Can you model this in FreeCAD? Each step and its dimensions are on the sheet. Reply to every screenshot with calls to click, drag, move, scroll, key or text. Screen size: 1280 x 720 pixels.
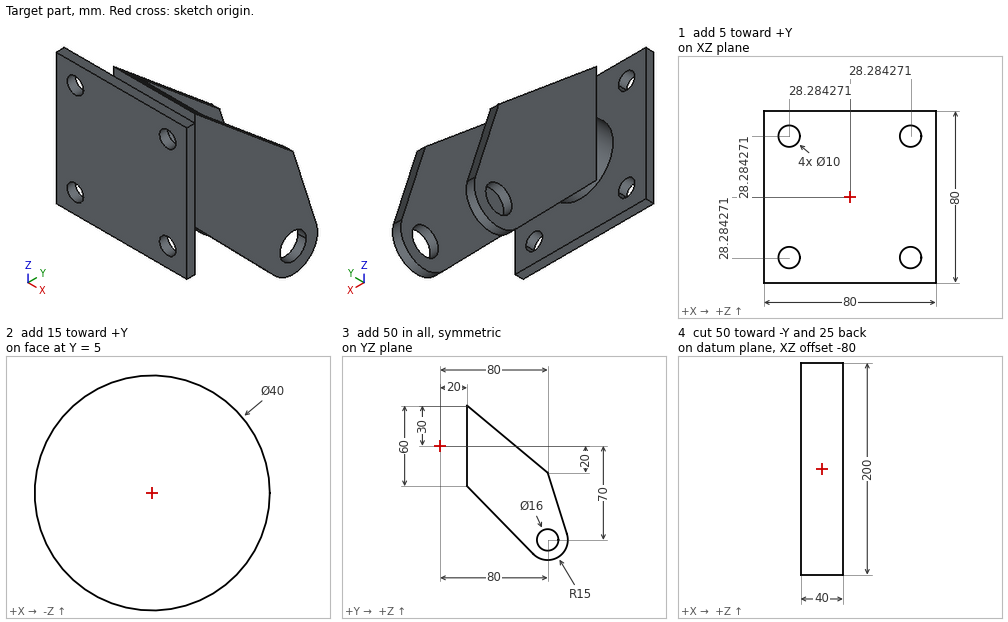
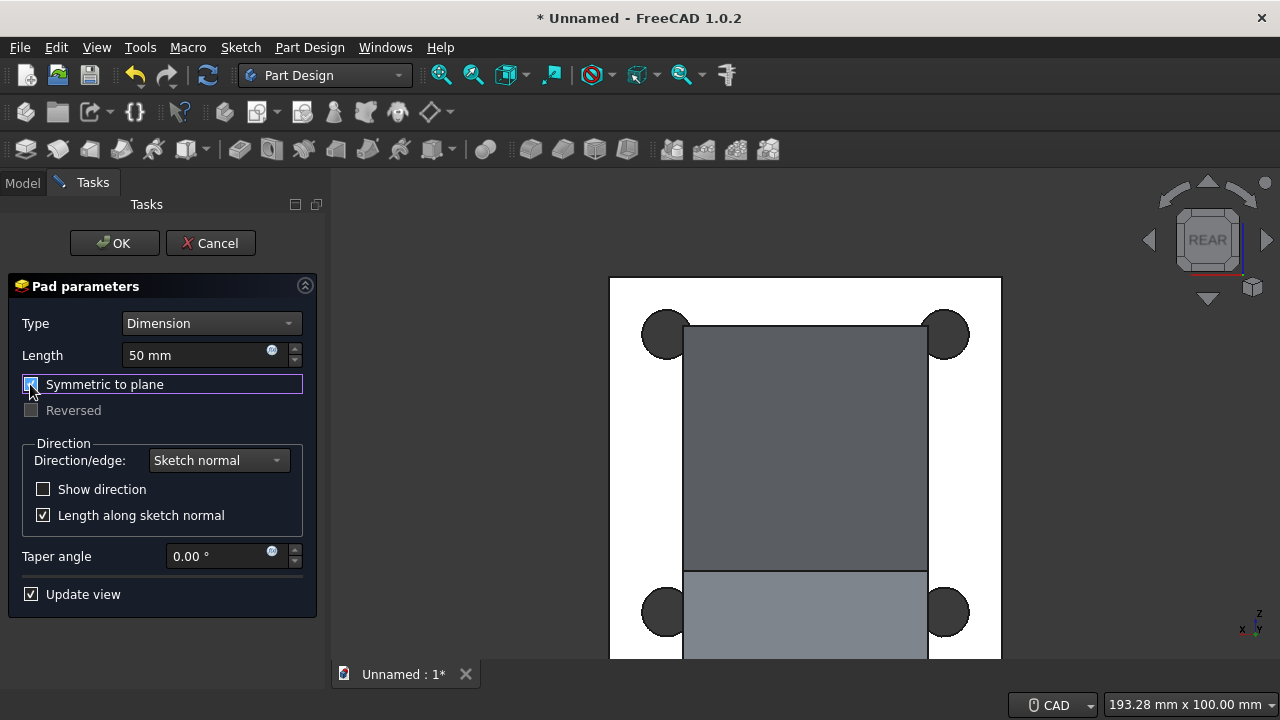
click(115, 243)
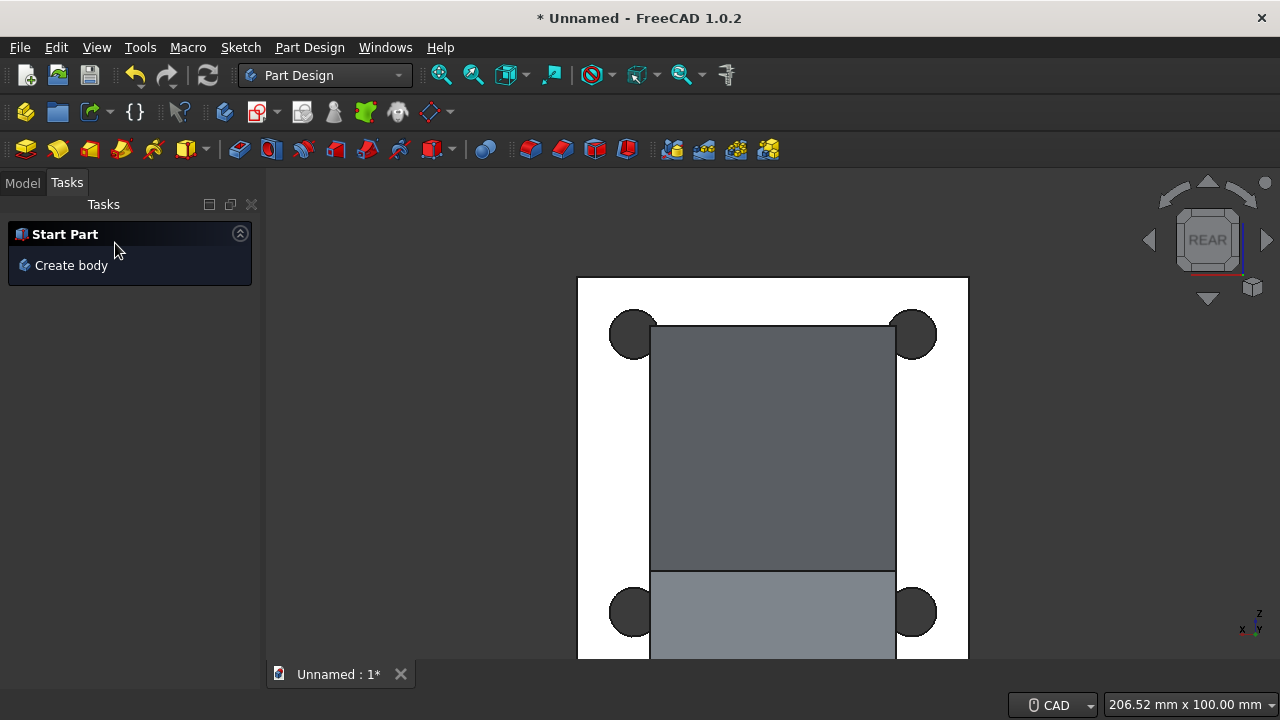
click(442, 76)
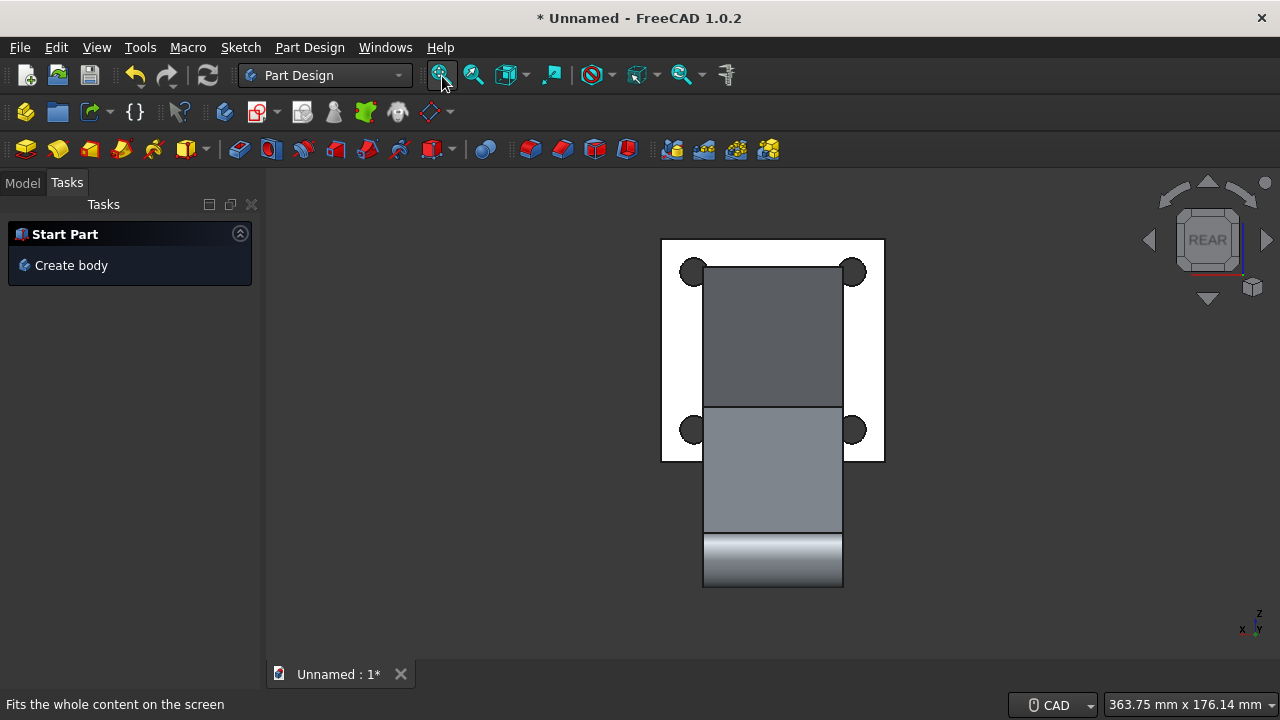
click(23, 182)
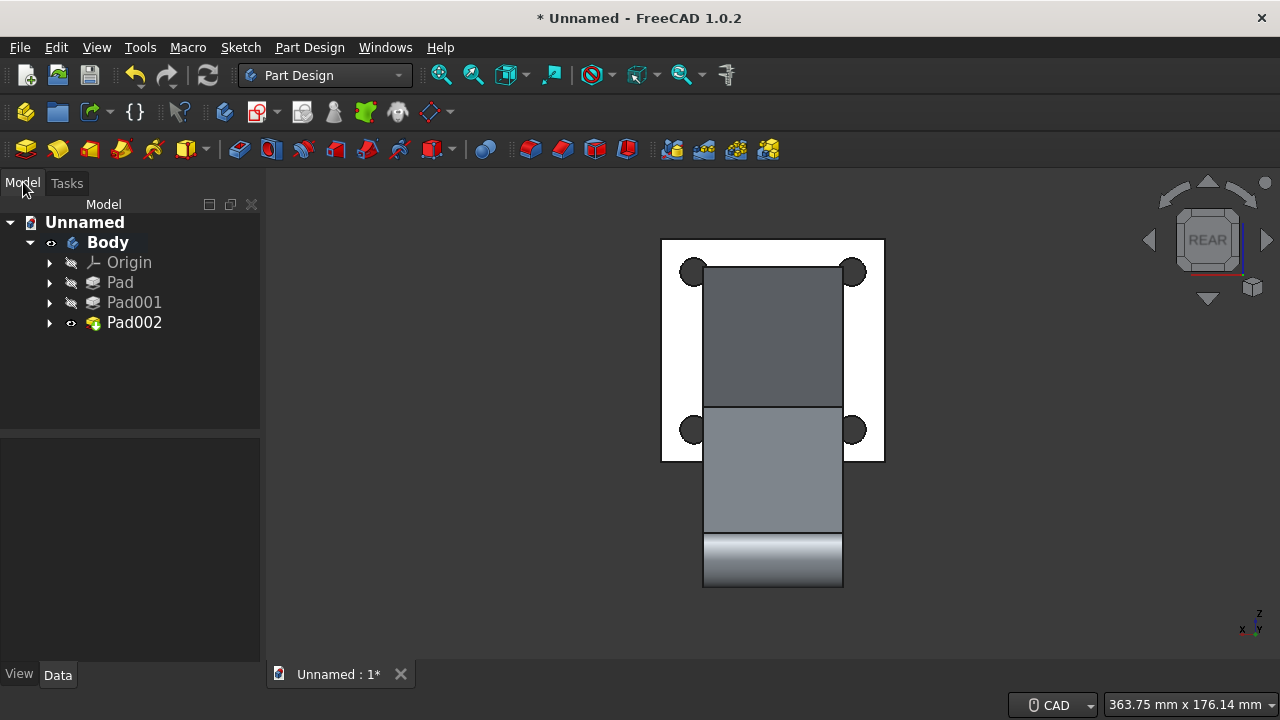
click(50, 263)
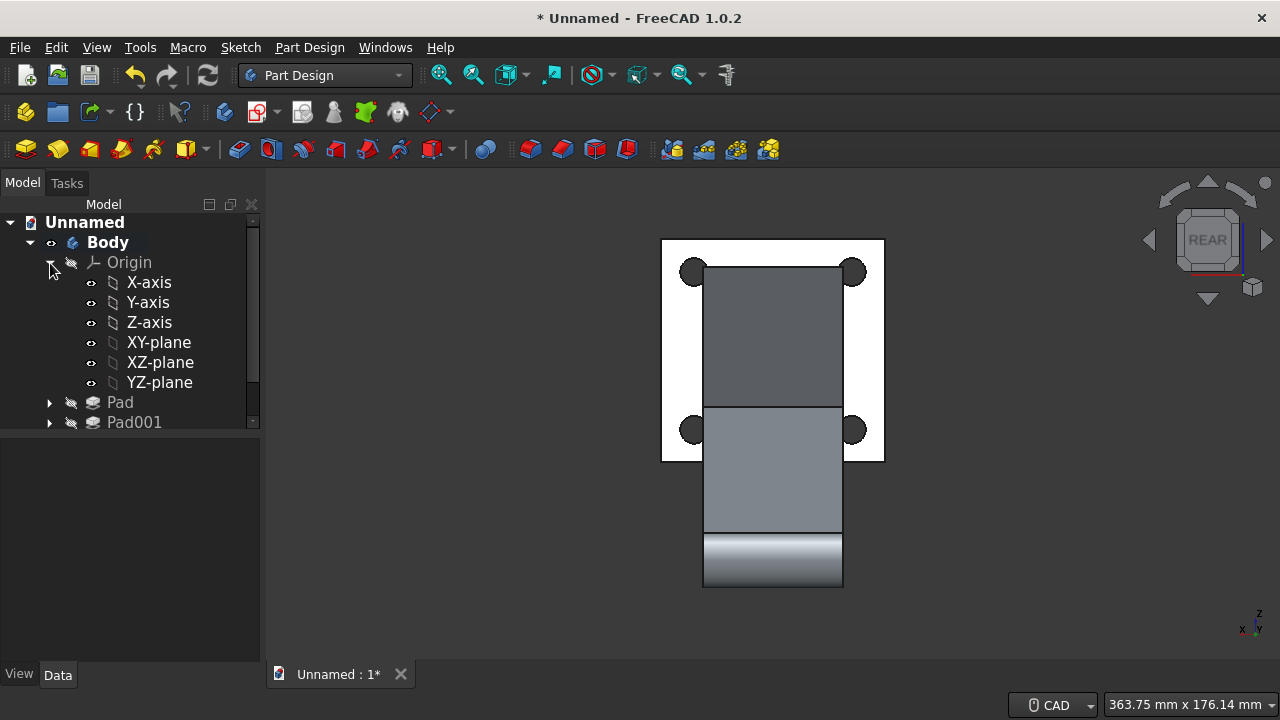
click(136, 363)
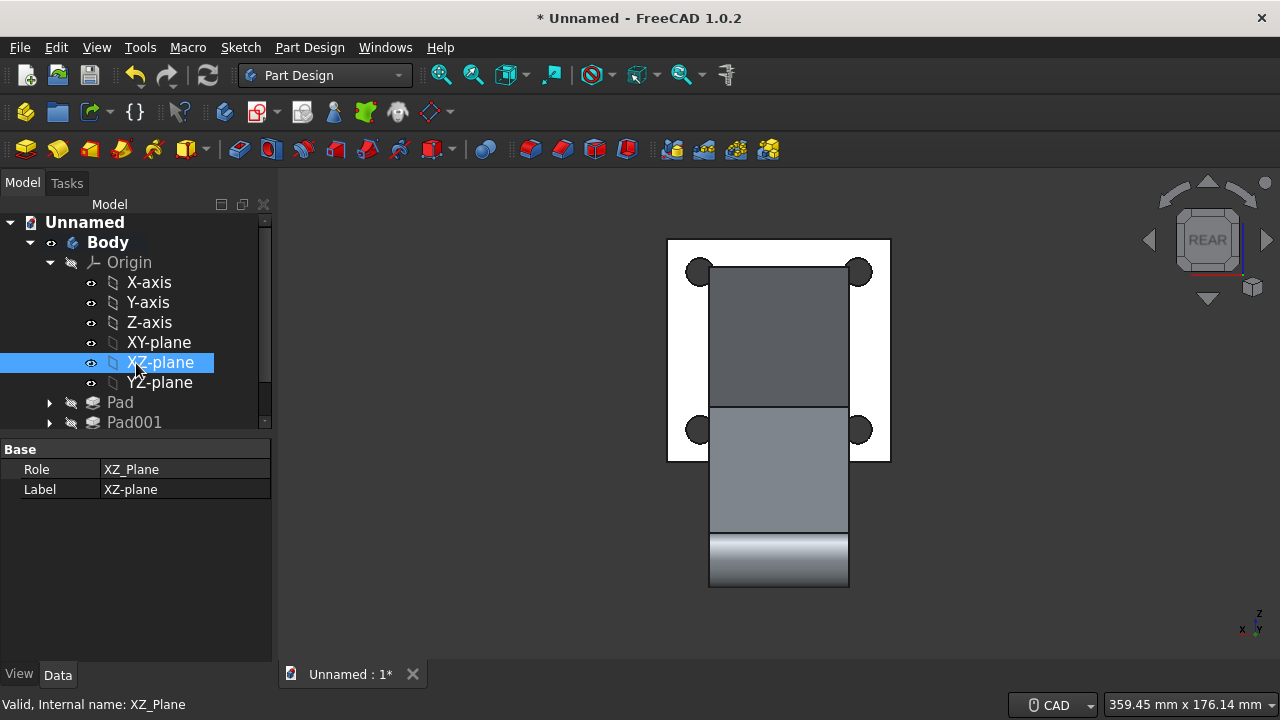
click(430, 112)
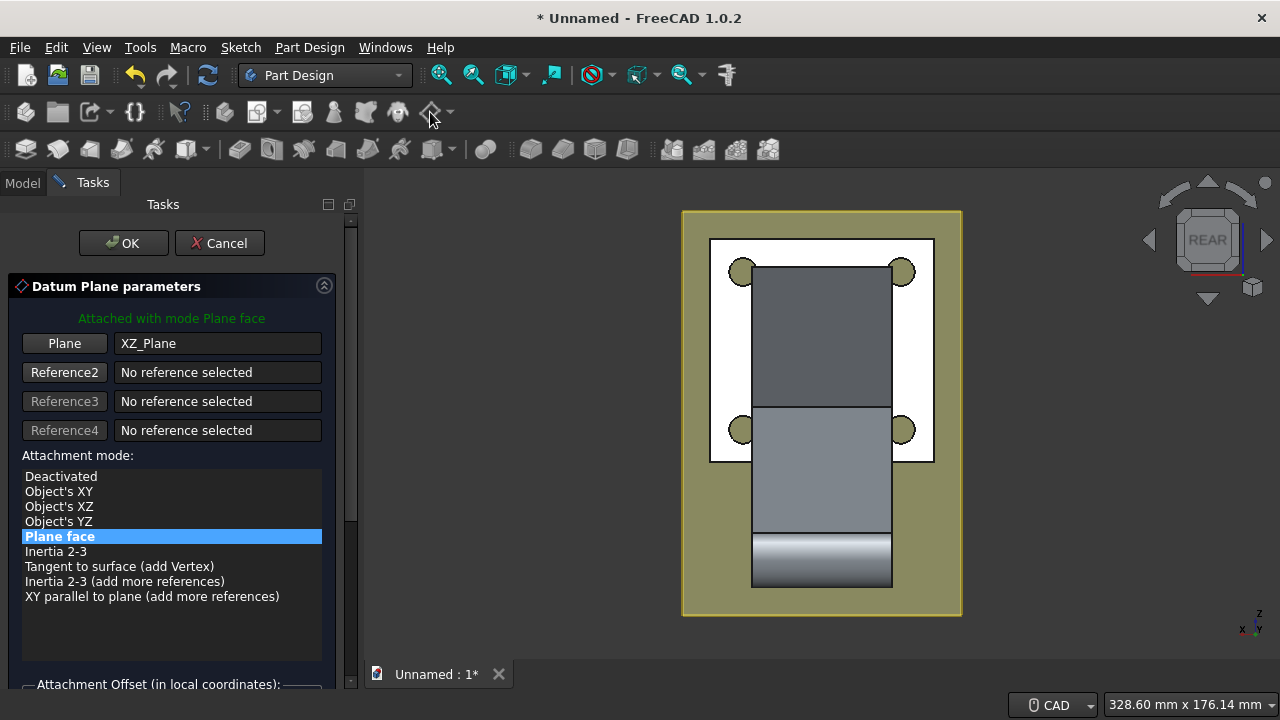
scroll(351, 451, down, 3)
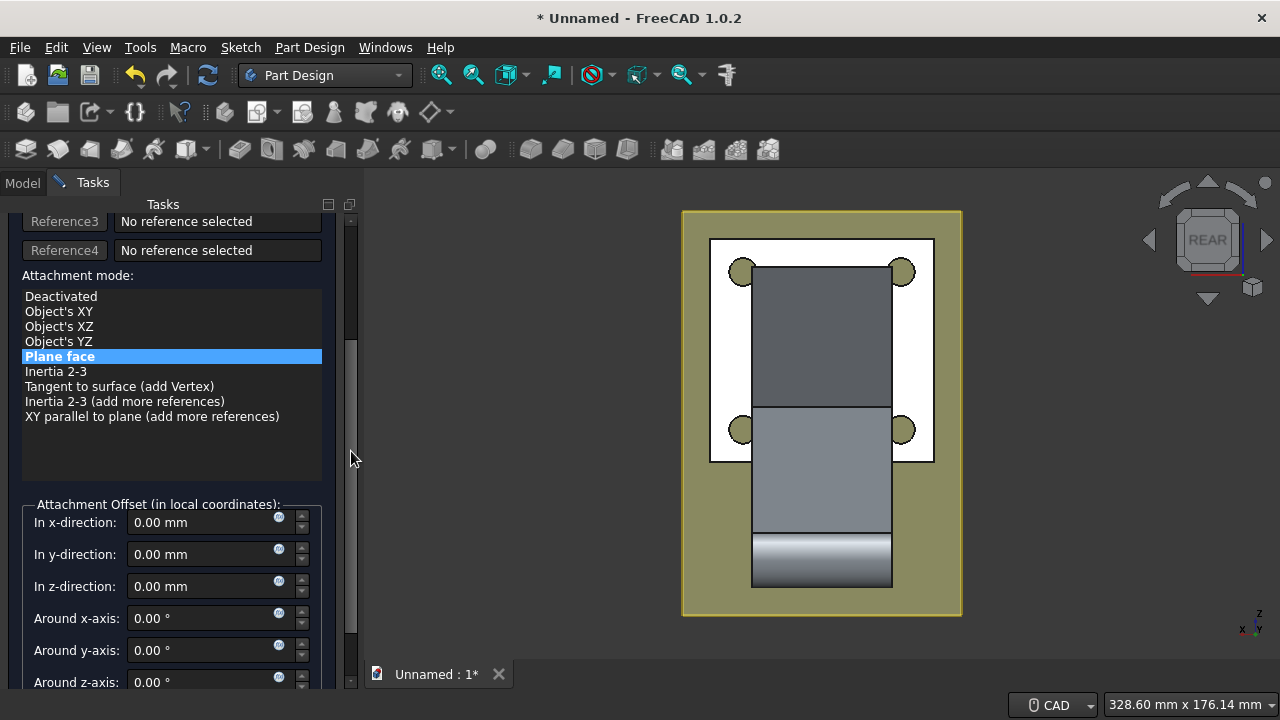
triple_click(210, 586)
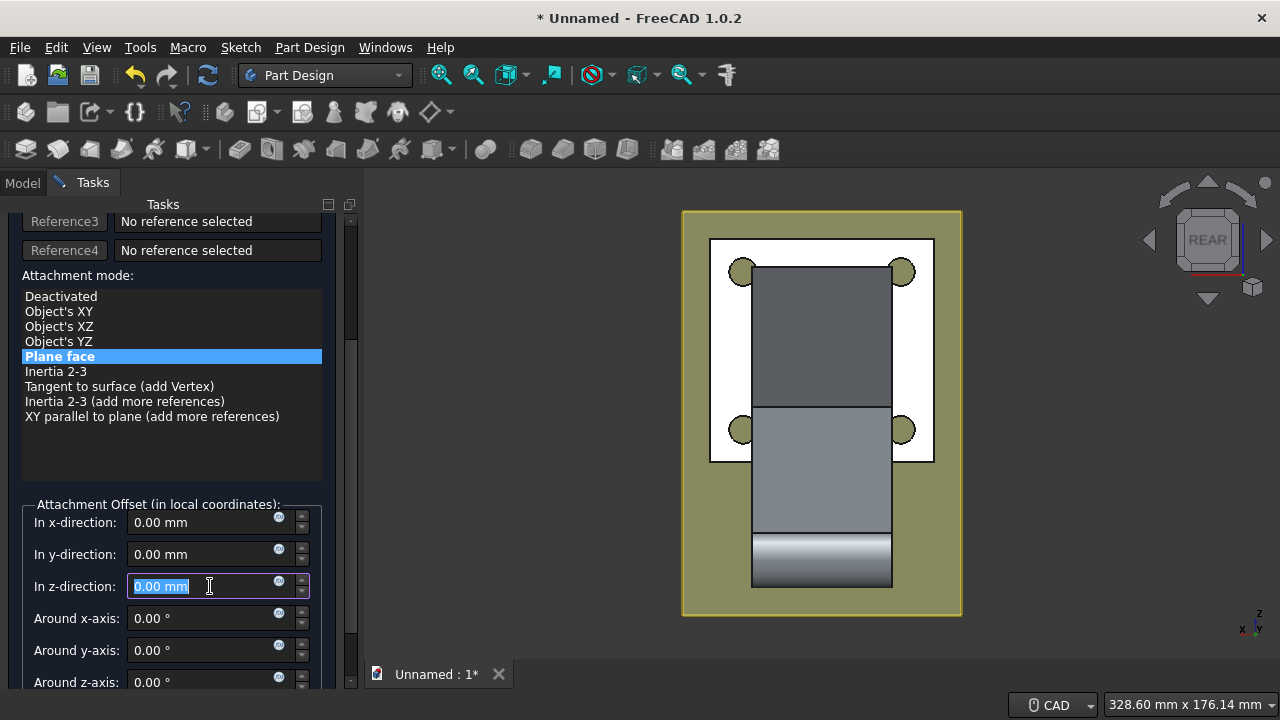
text(-80)
key(Tab)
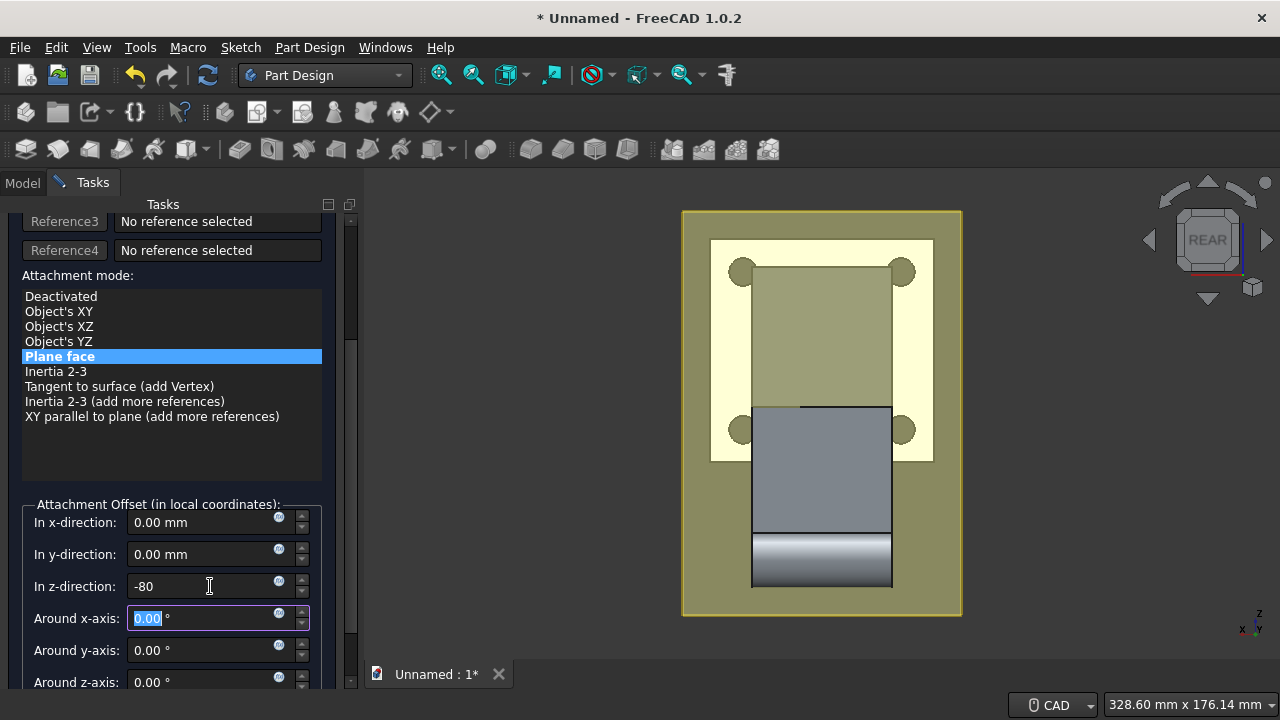
scroll(351, 451, up, 4)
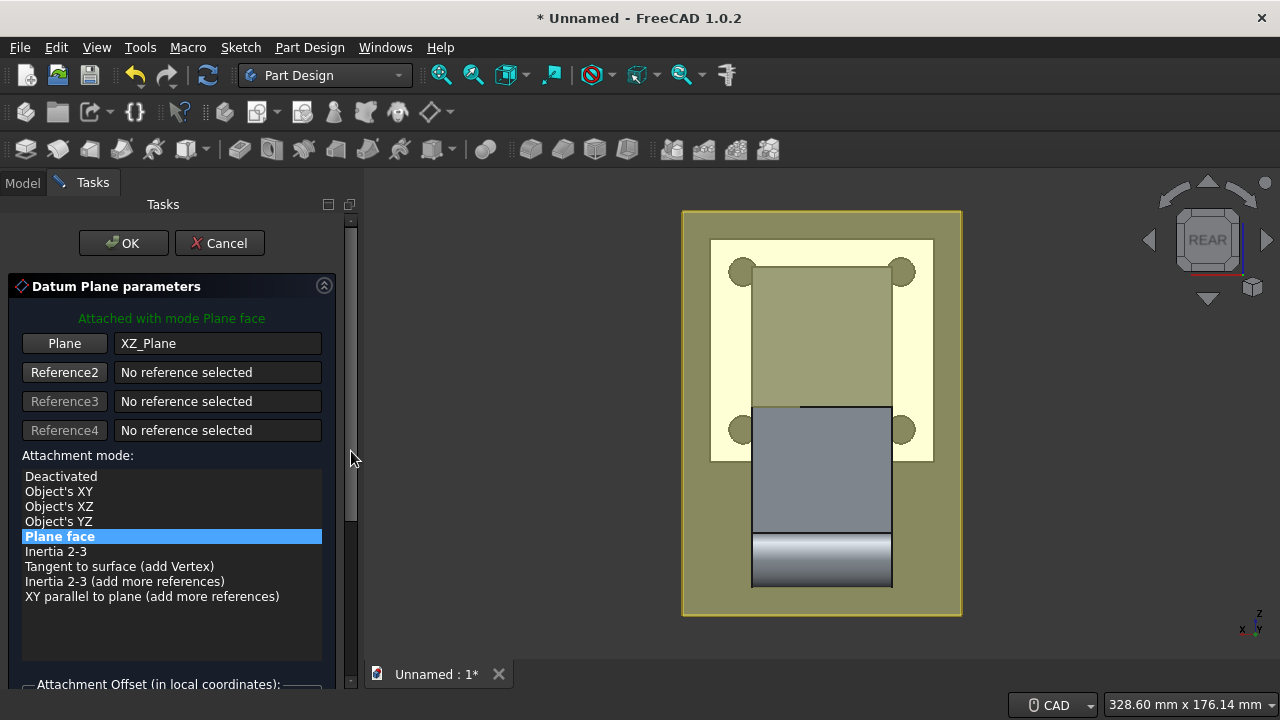
click(124, 243)